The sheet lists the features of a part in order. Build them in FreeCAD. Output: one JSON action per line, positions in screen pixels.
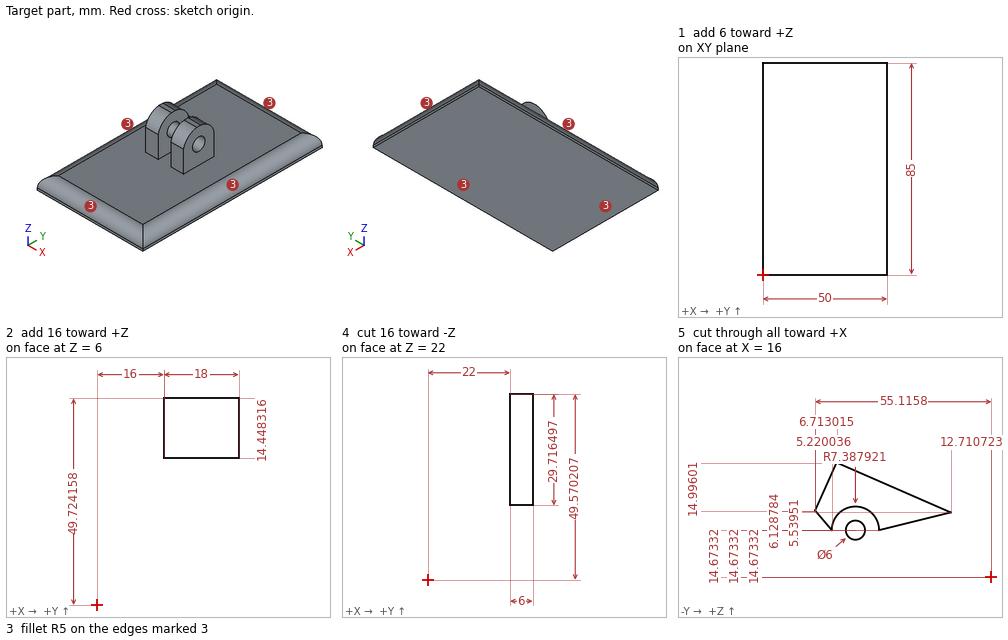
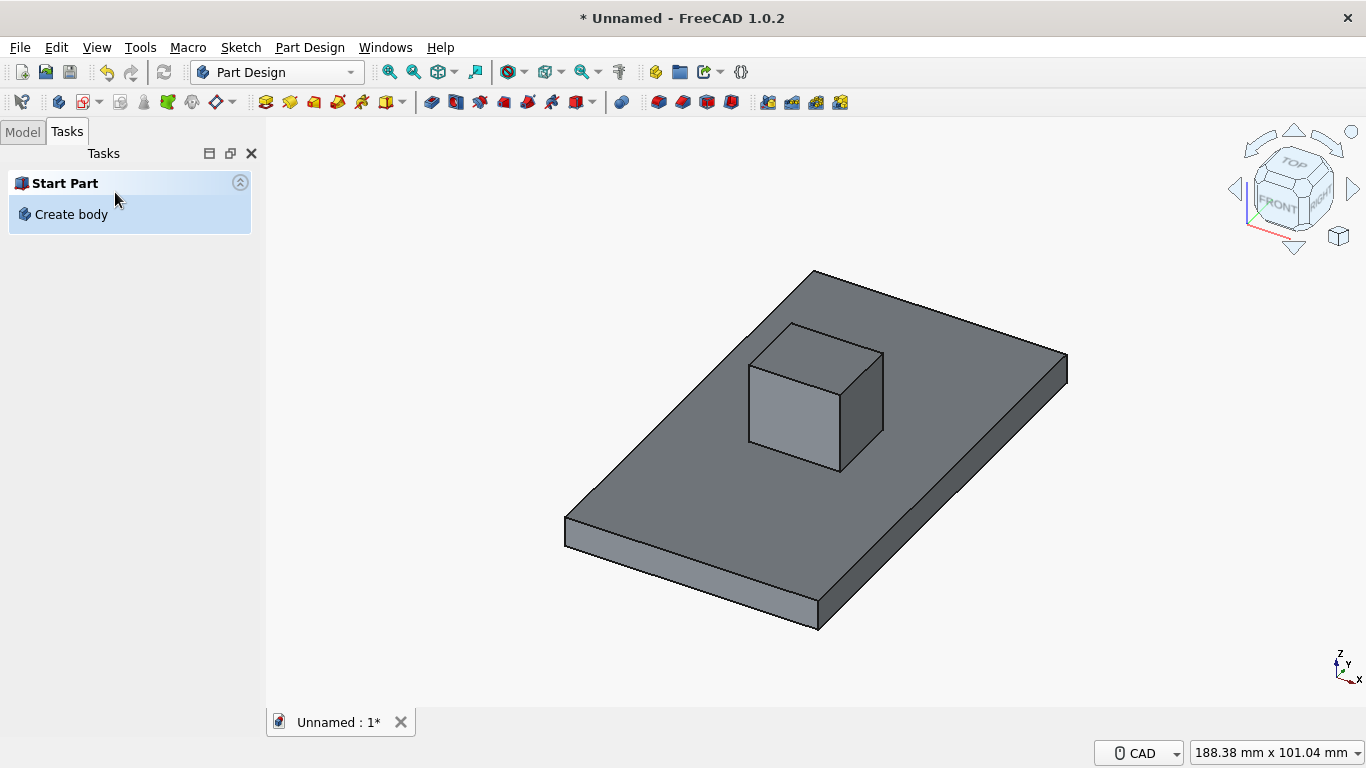
{"action": "left_click", "coordinate": [942, 477]}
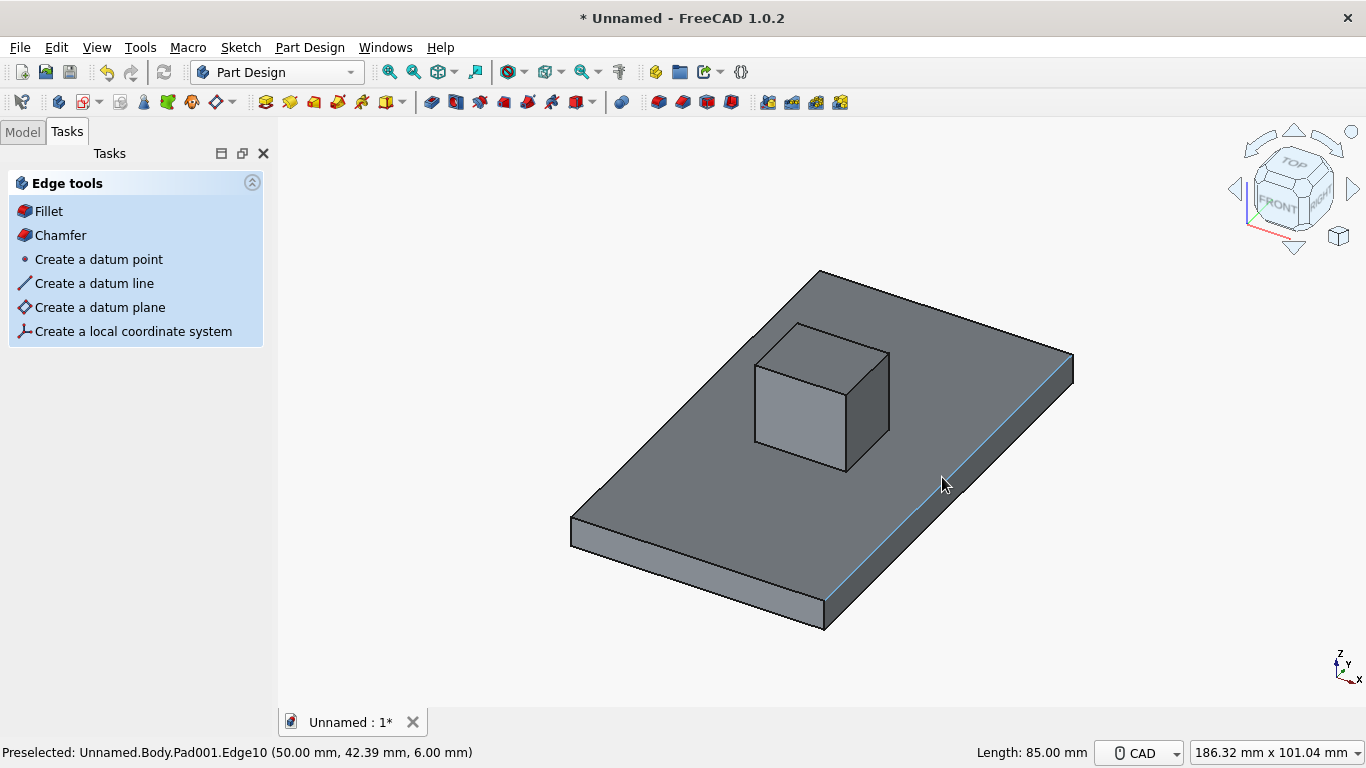
{"action": "left_click", "coordinate": [698, 558], "text": "ctrl"}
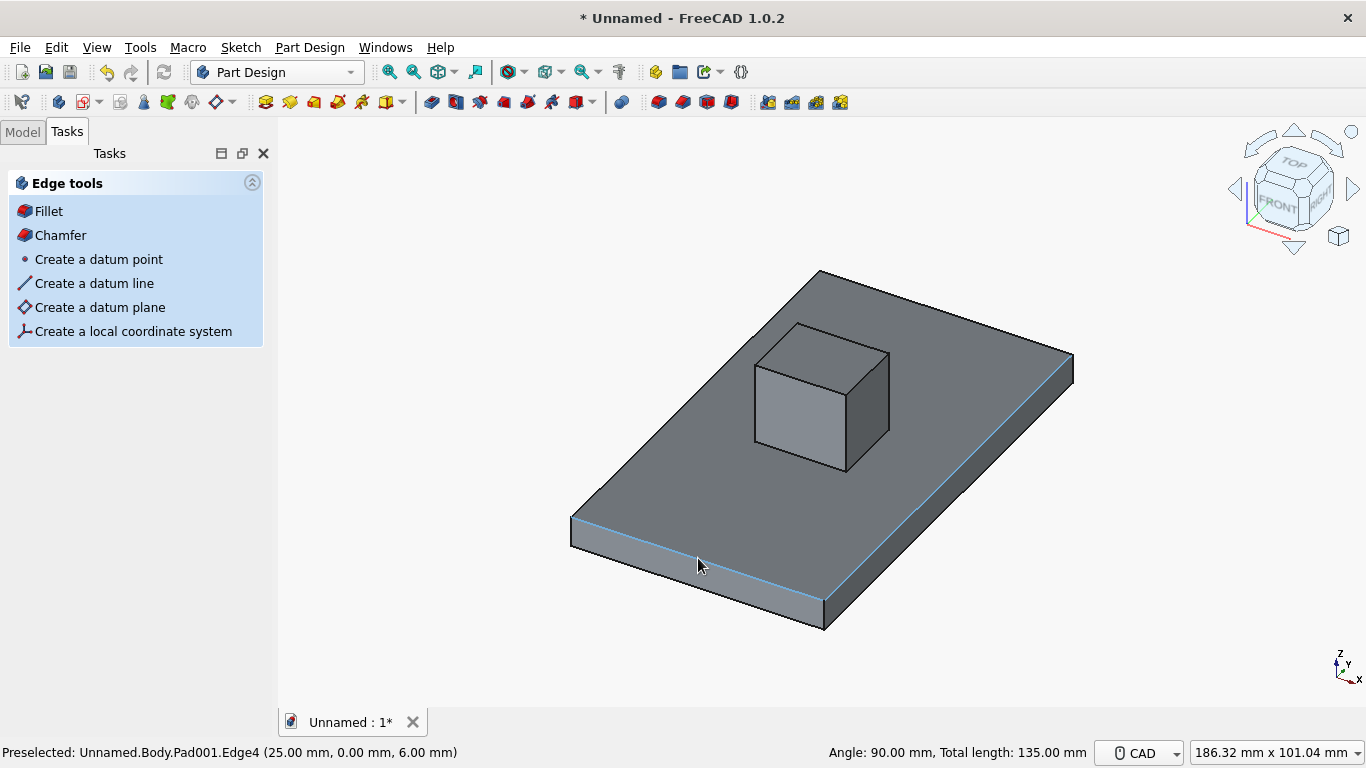
{"action": "key", "text": "0"}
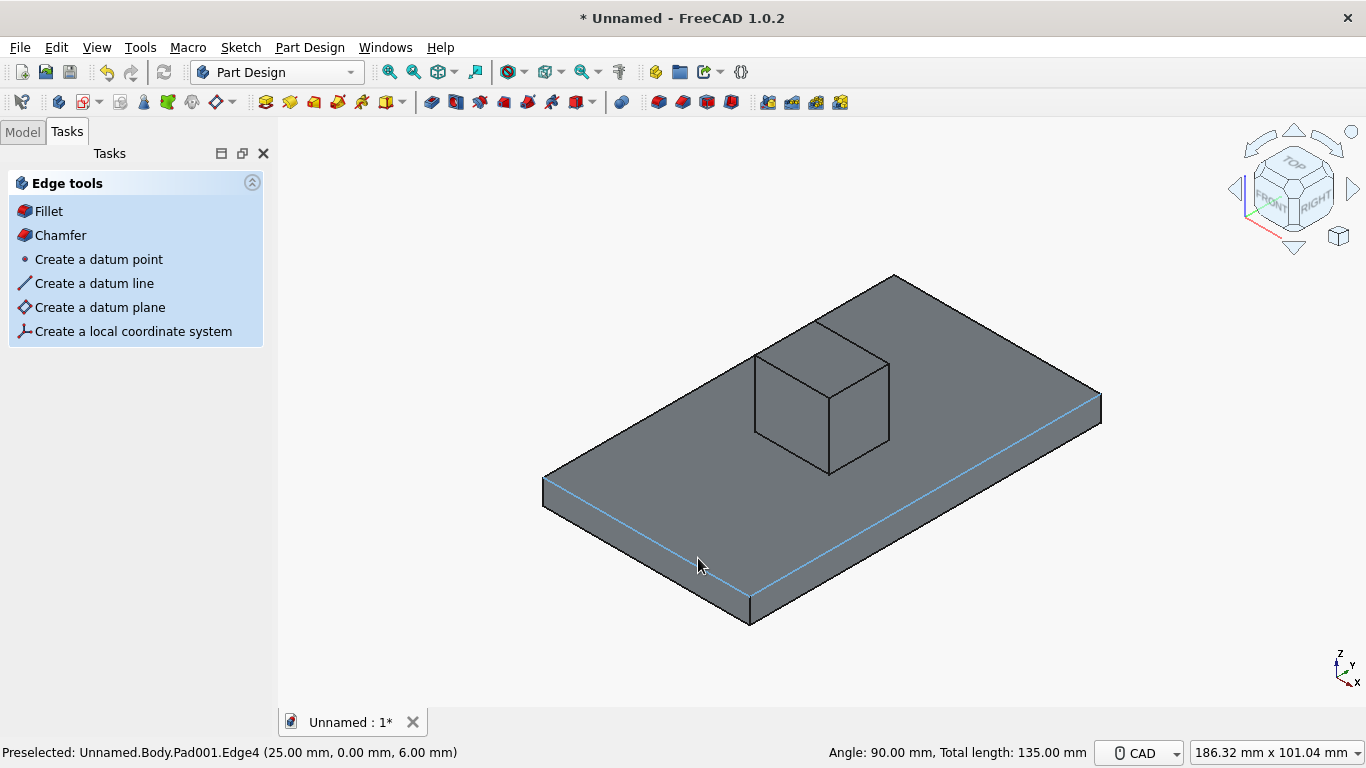
{"action": "key", "text": "2"}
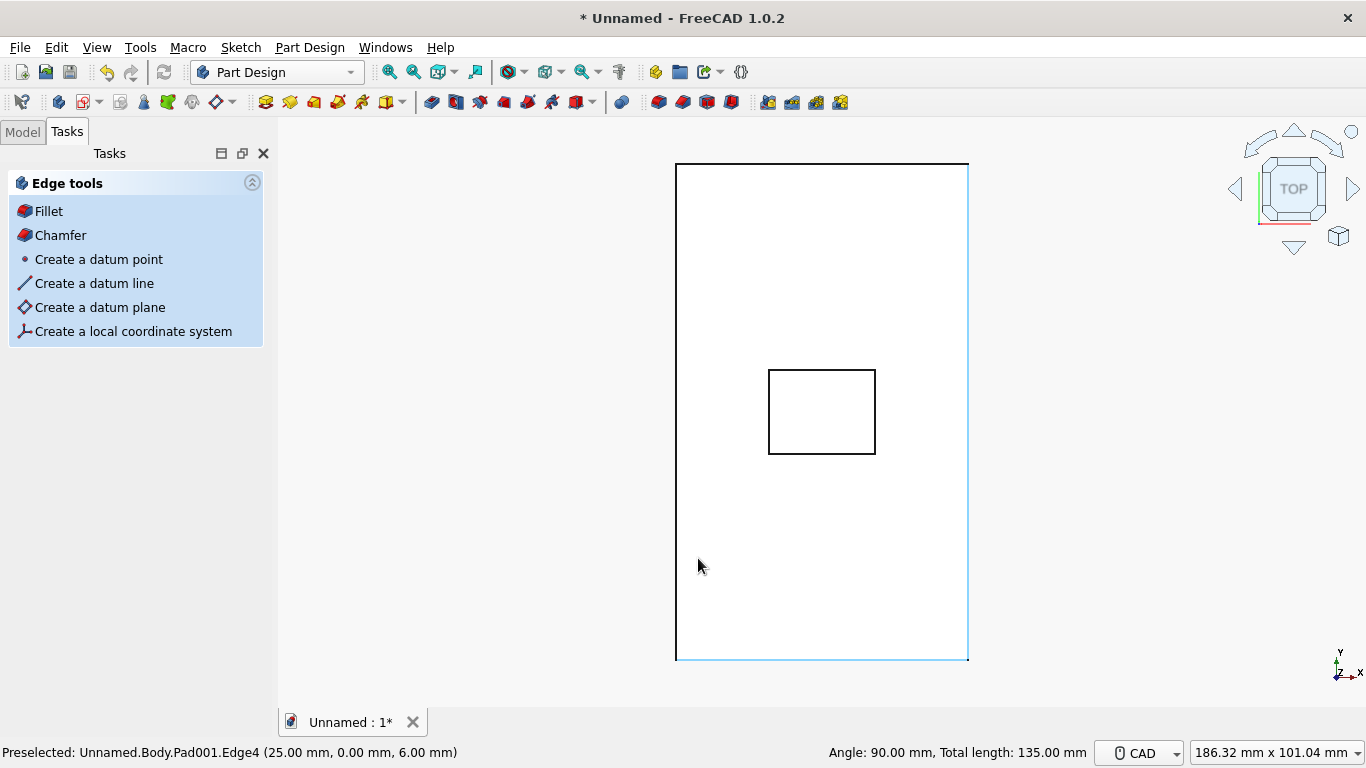
{"action": "left_click", "coordinate": [822, 163], "text": "ctrl"}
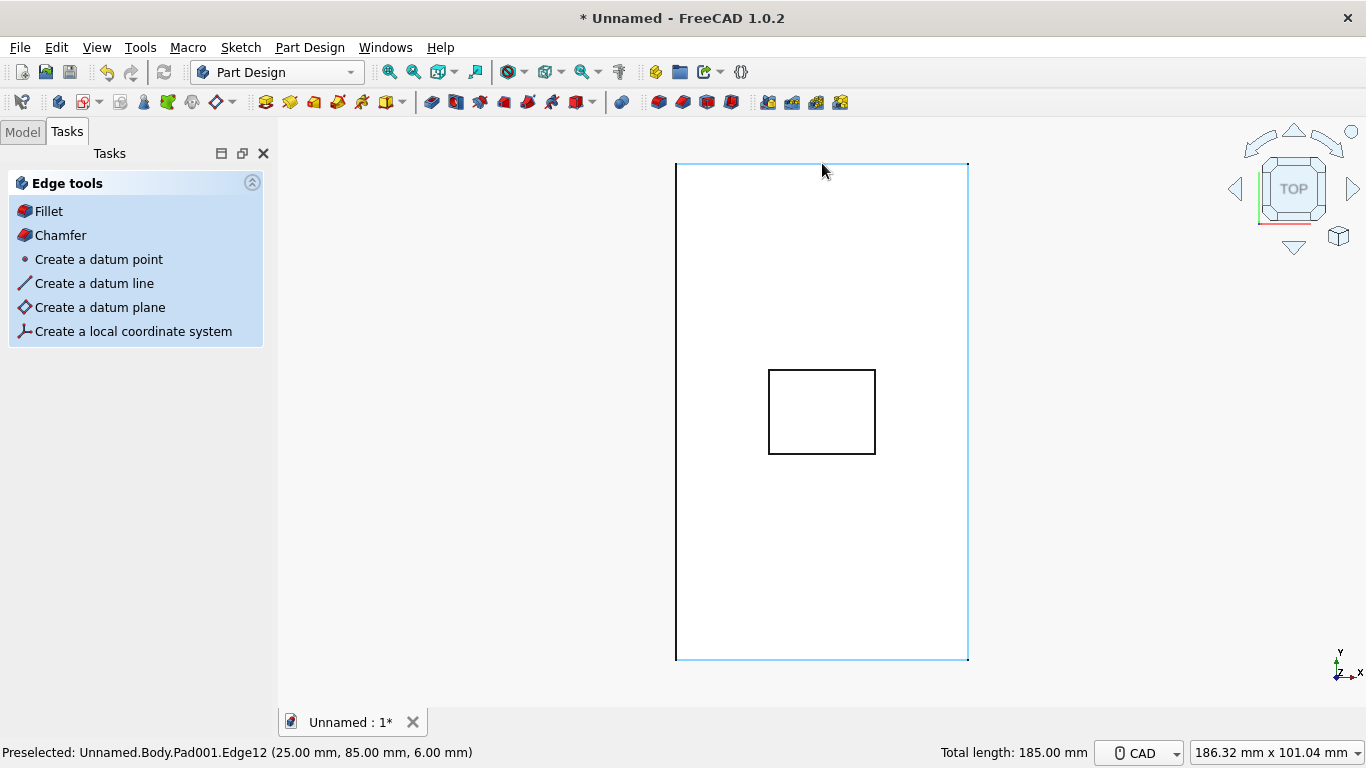
{"action": "left_click", "coordinate": [676, 411], "text": "ctrl"}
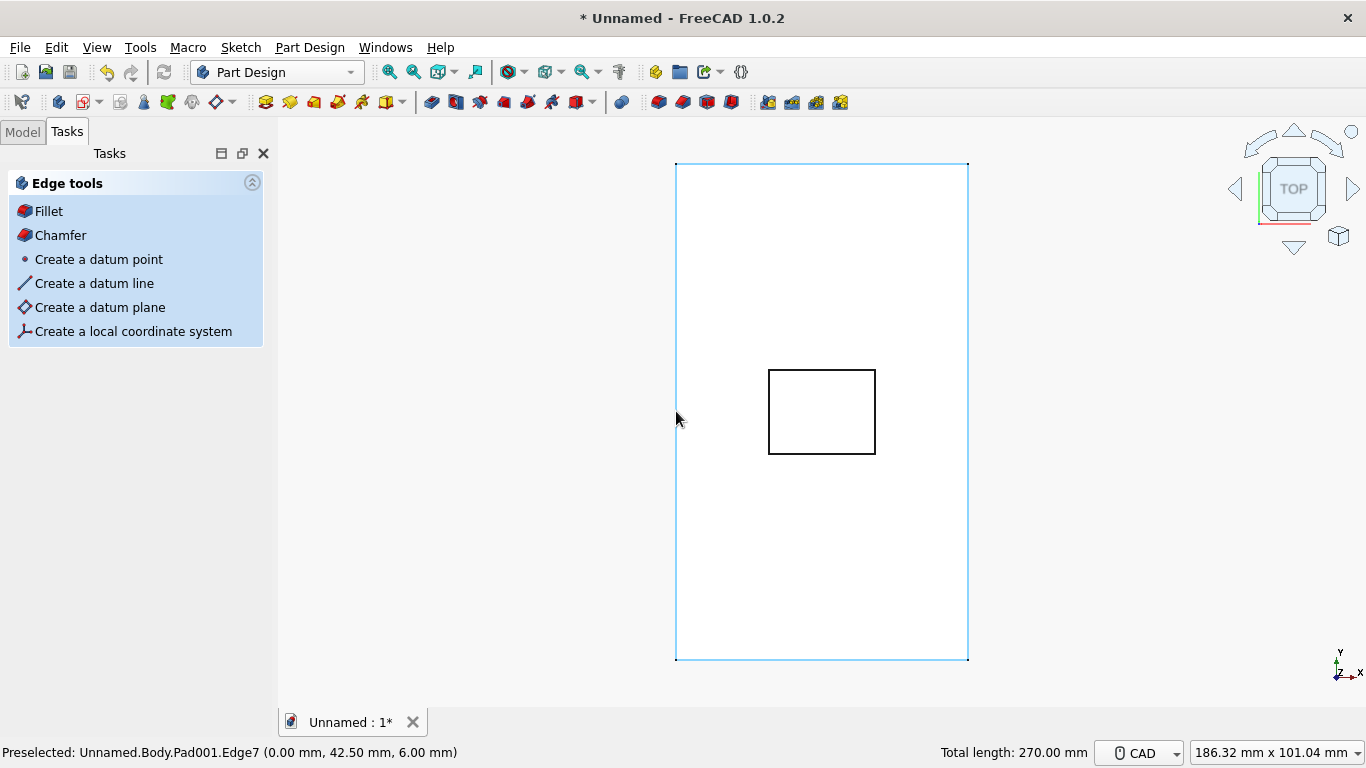
{"action": "left_click", "coordinate": [660, 102]}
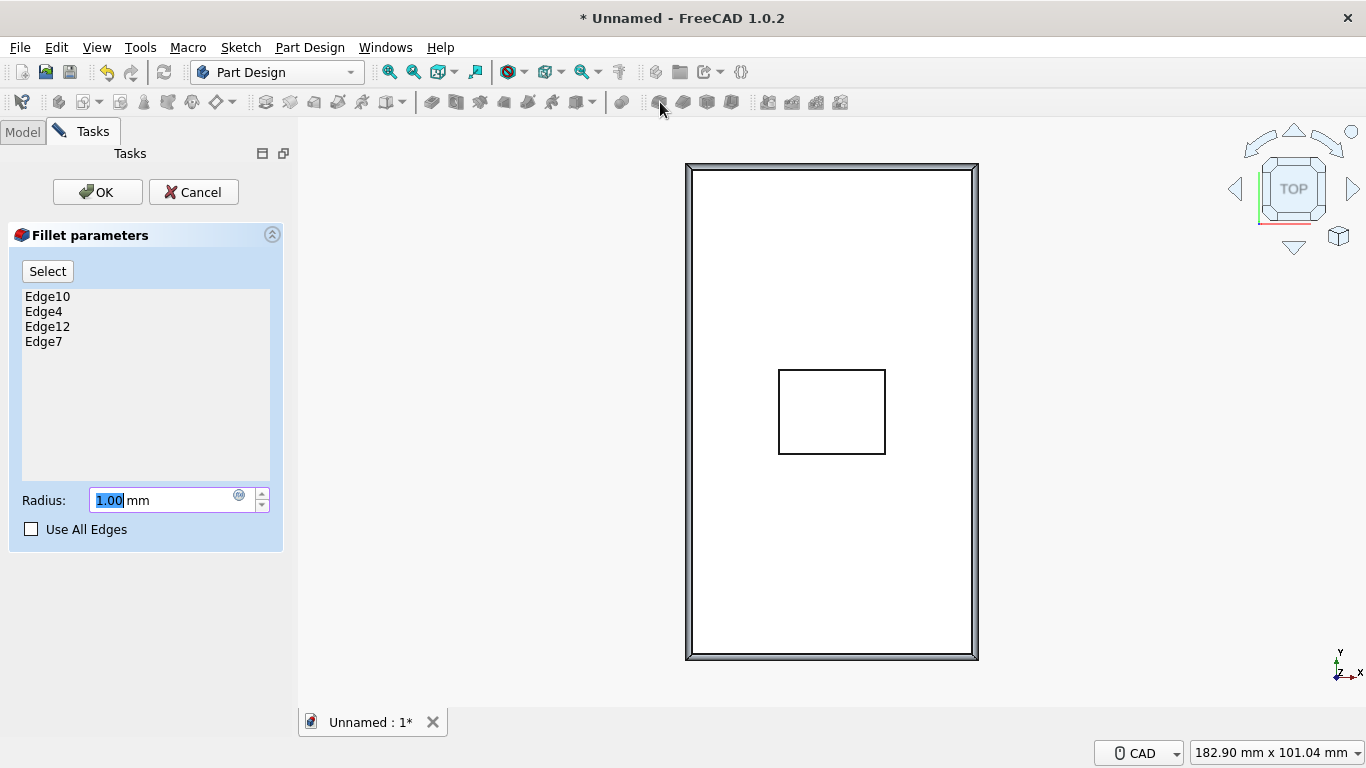
{"action": "type", "text": "5"}
{"action": "key", "text": "Tab"}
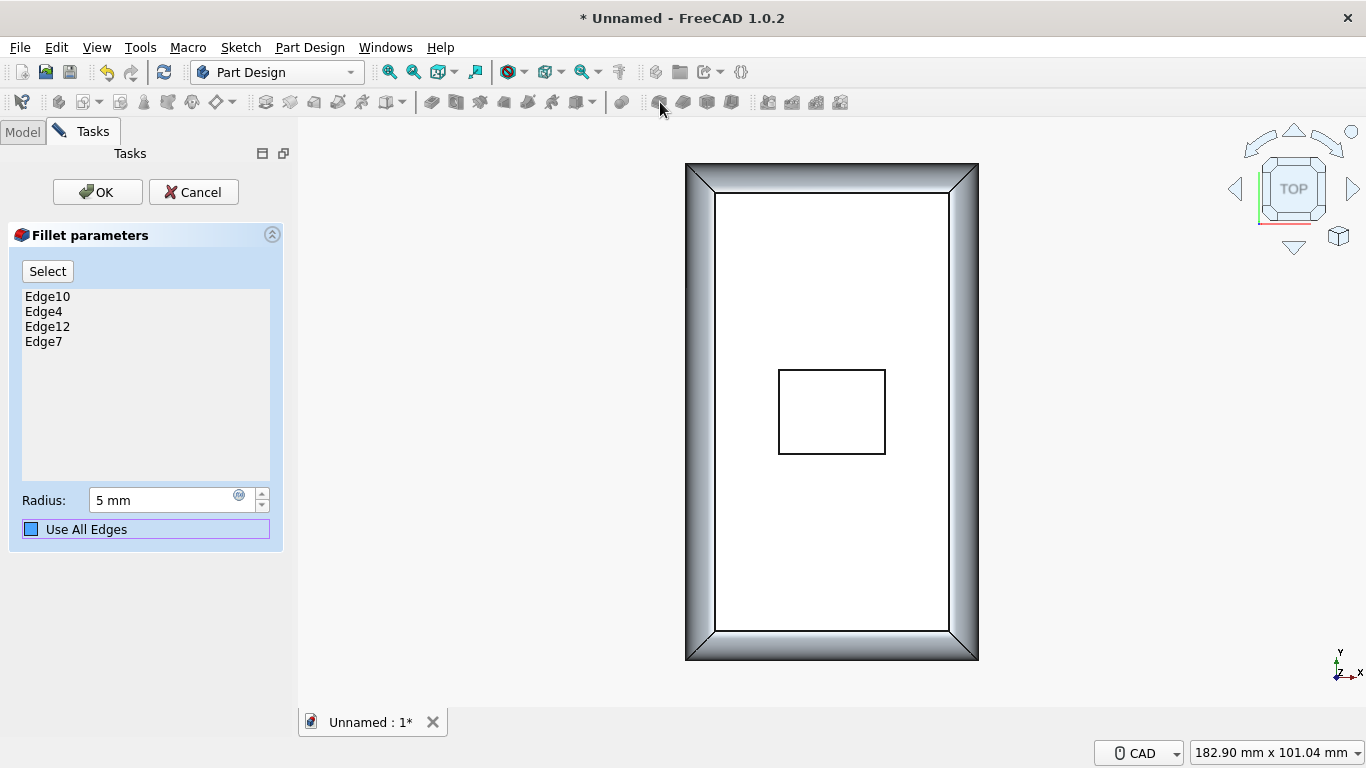
{"action": "left_click", "coordinate": [98, 192]}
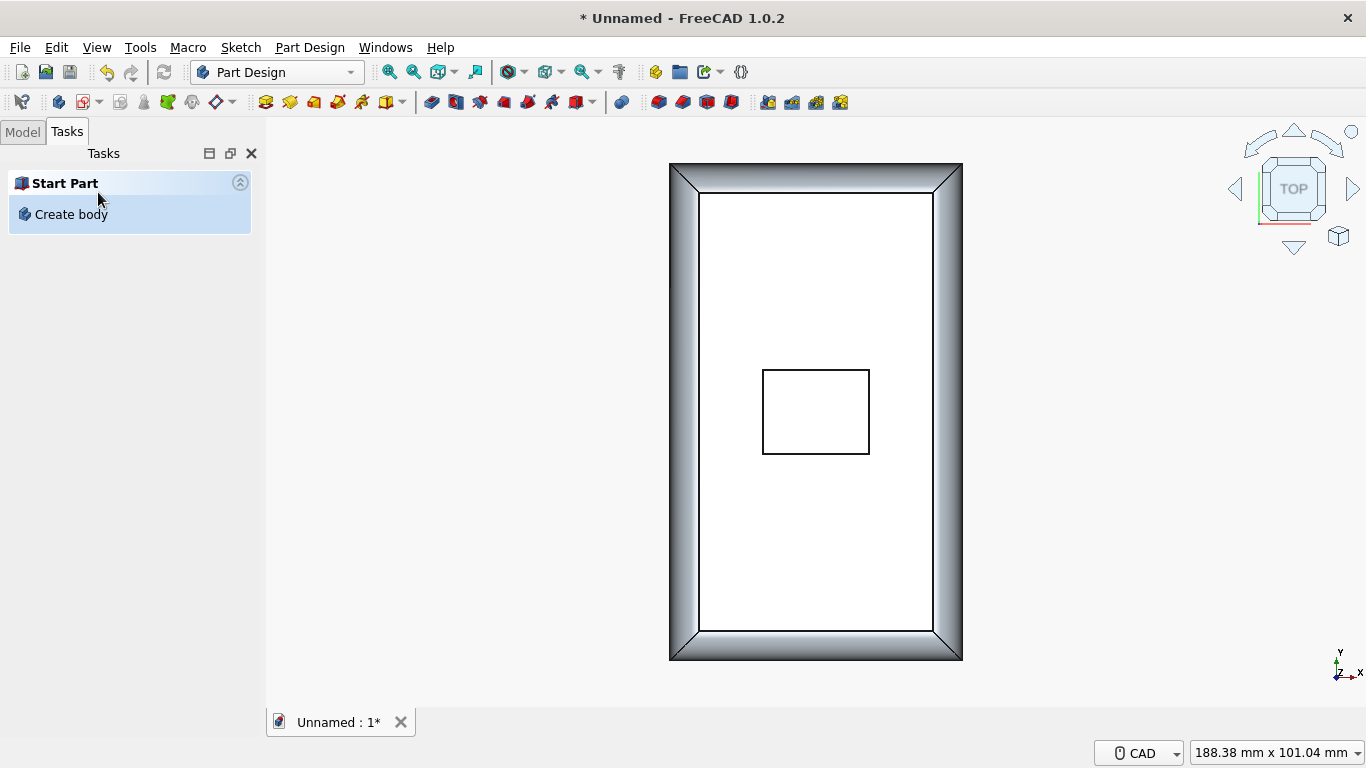
{"action": "left_click", "coordinate": [816, 411]}